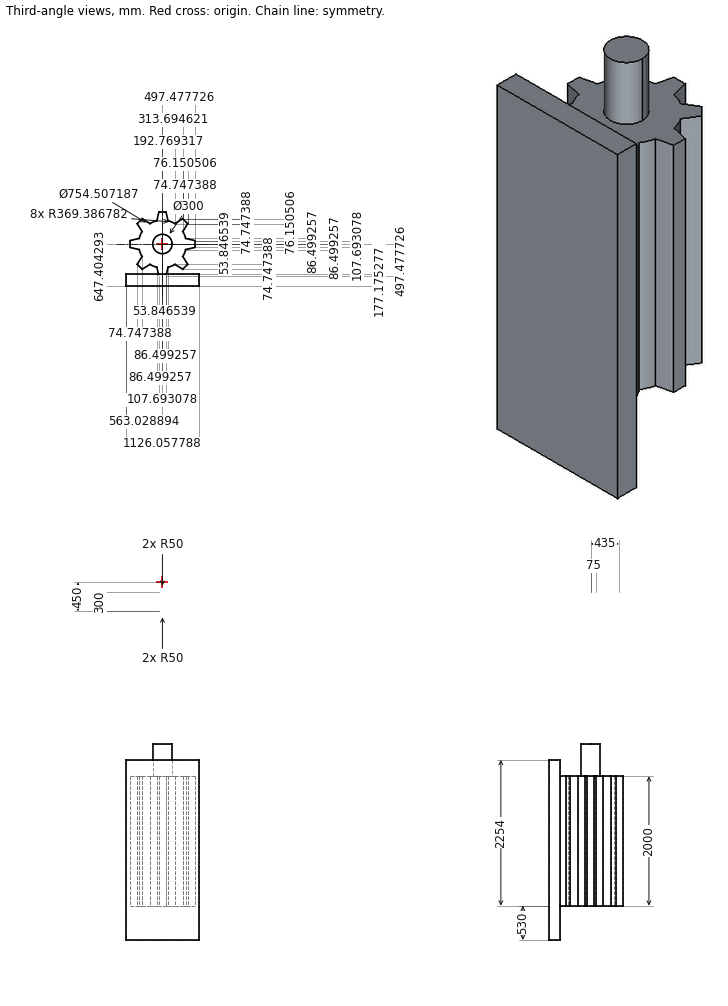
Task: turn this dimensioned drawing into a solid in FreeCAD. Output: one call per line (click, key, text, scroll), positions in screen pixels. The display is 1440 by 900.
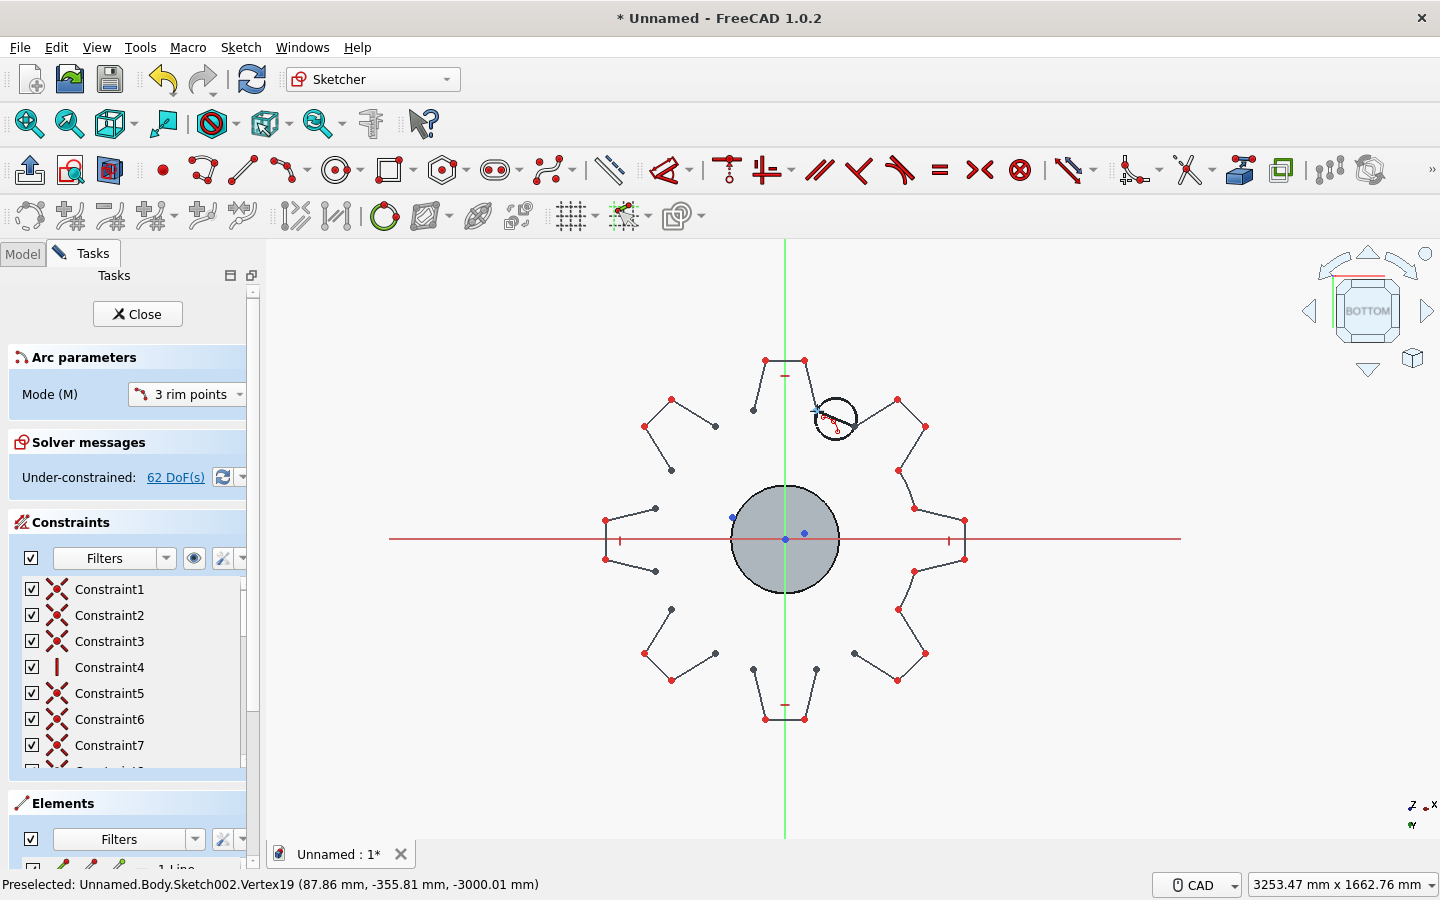
scroll(836, 416, up, 12)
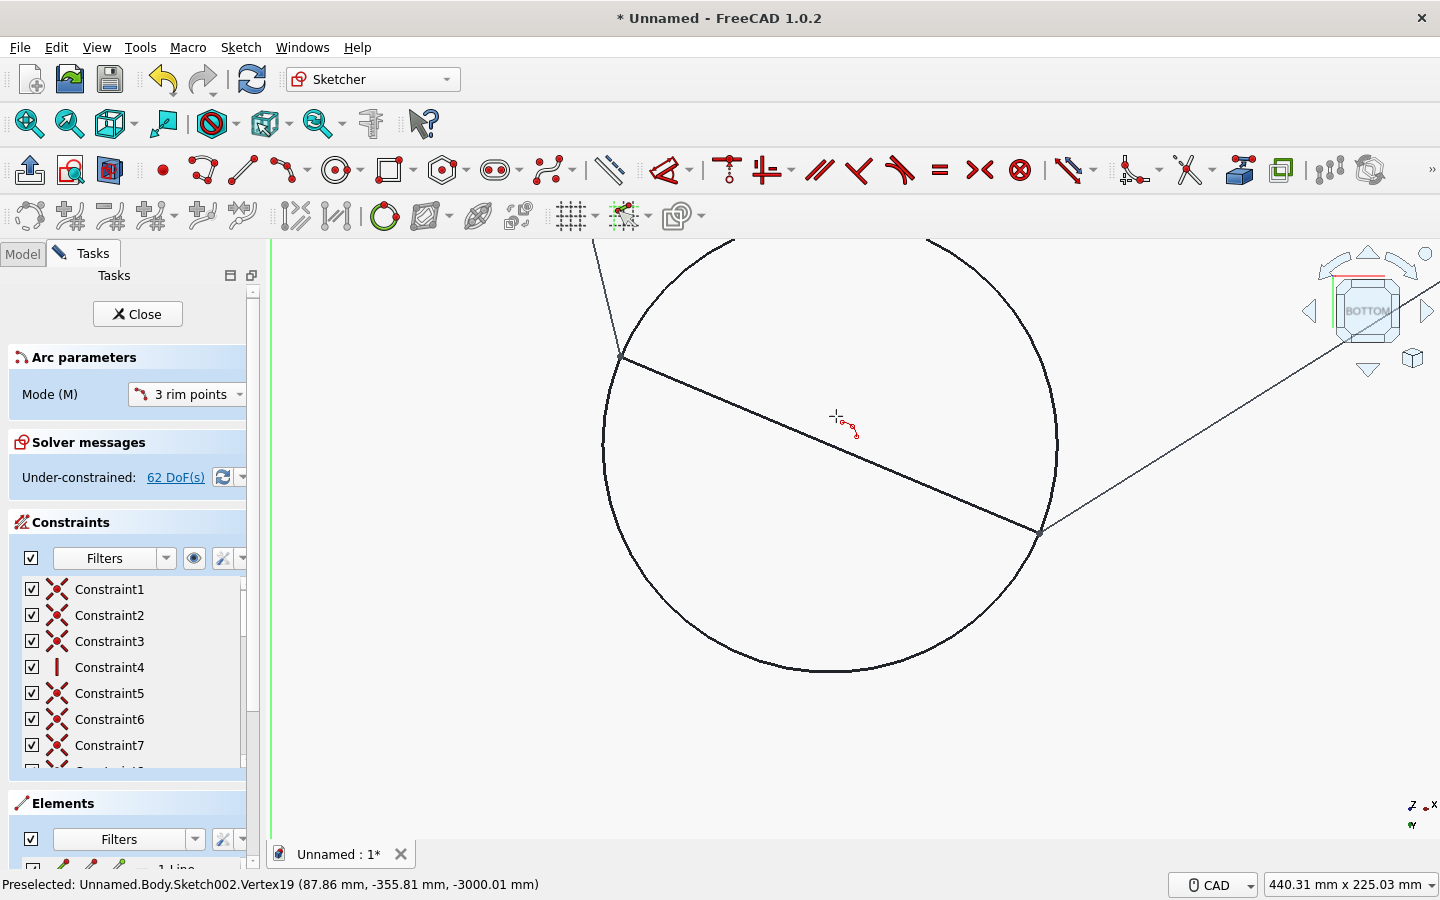
click(833, 415)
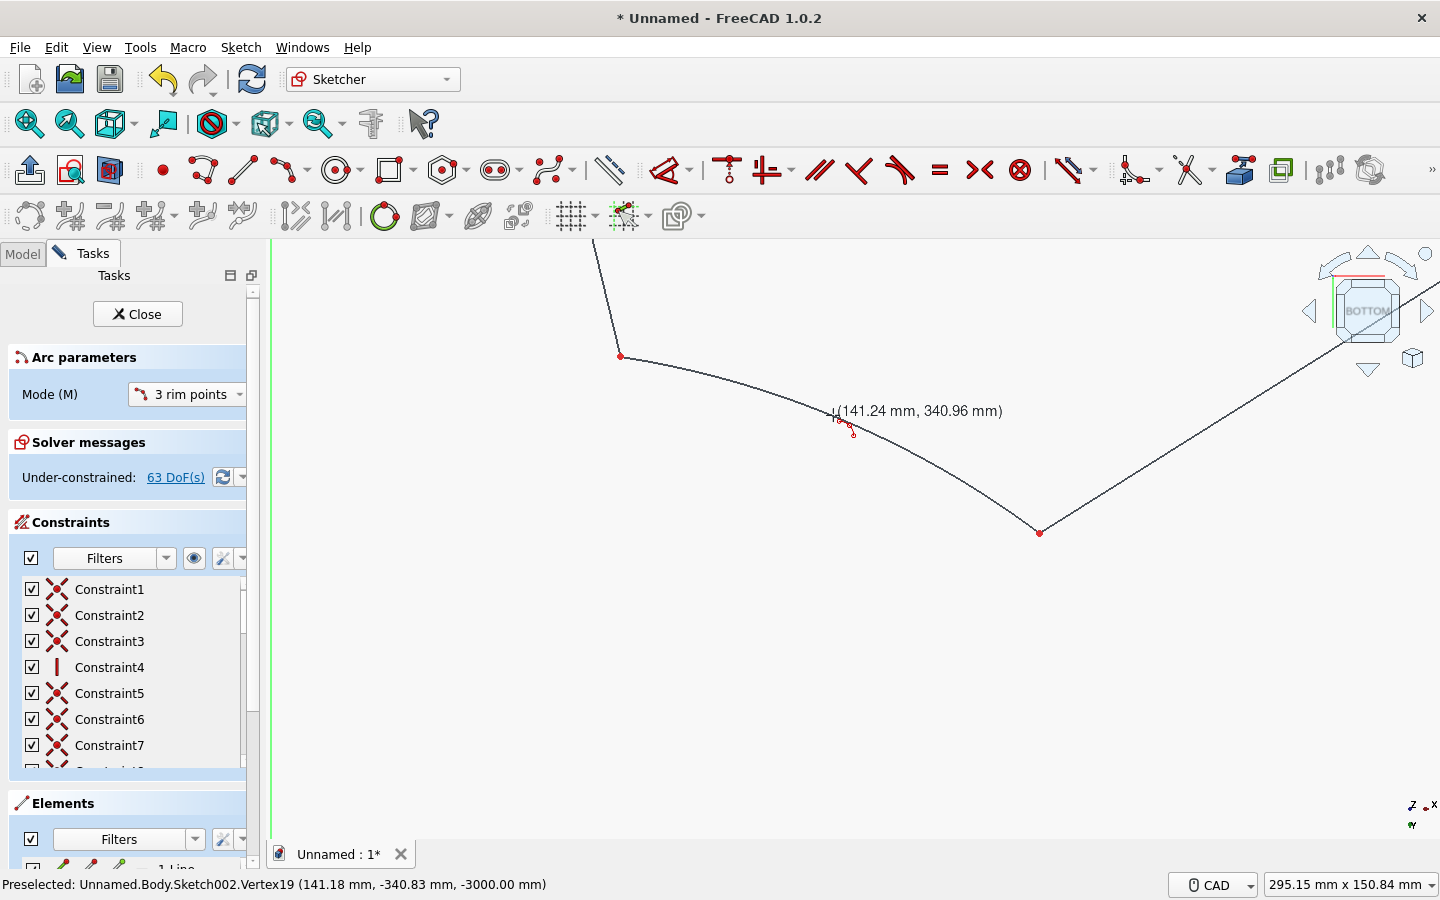
scroll(836, 416, down, 12)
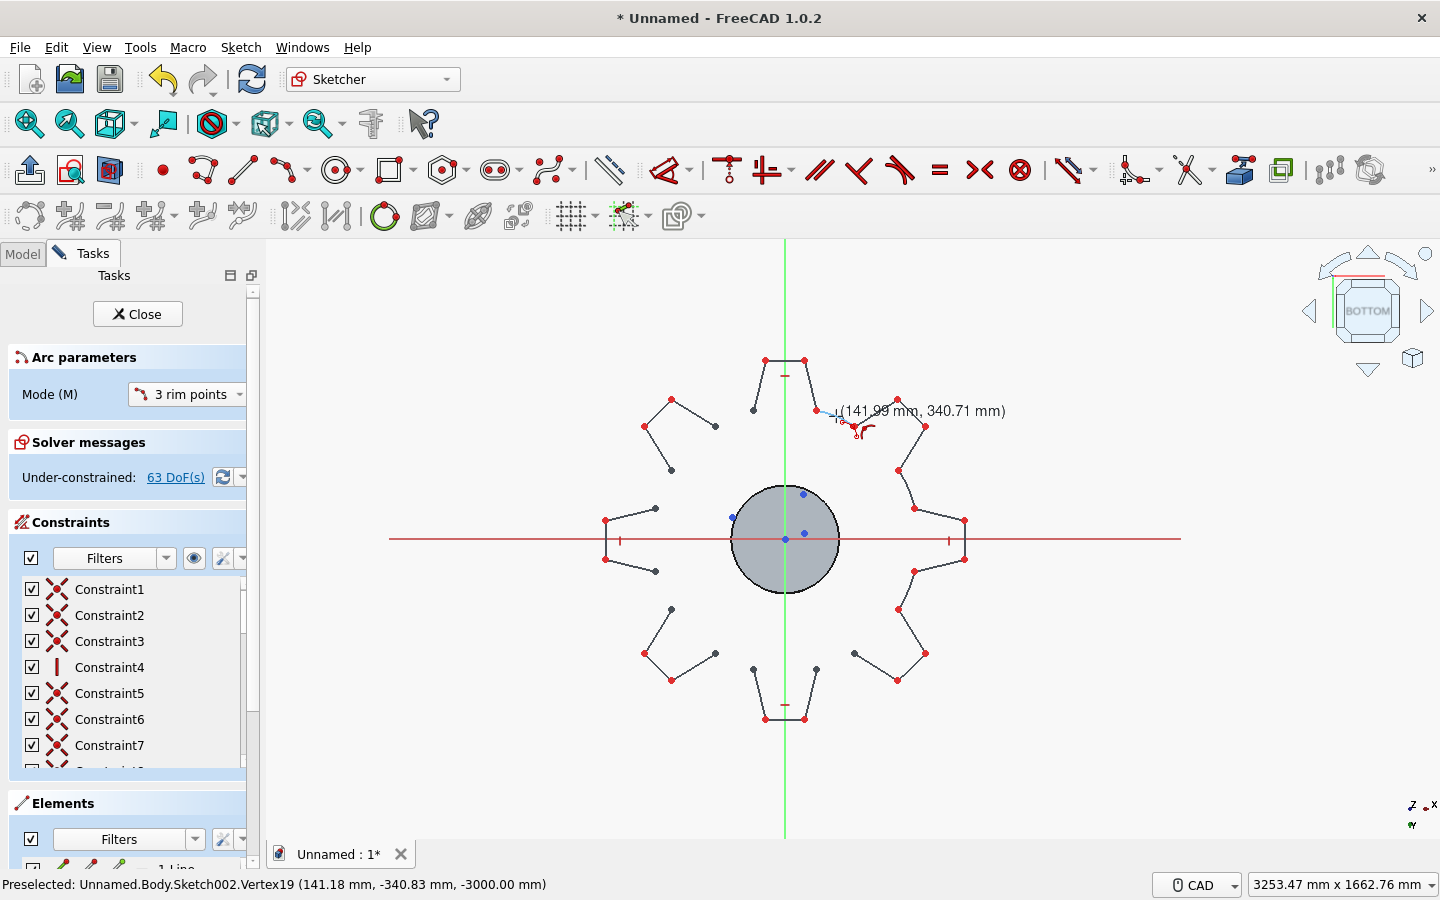
click(754, 411)
click(716, 427)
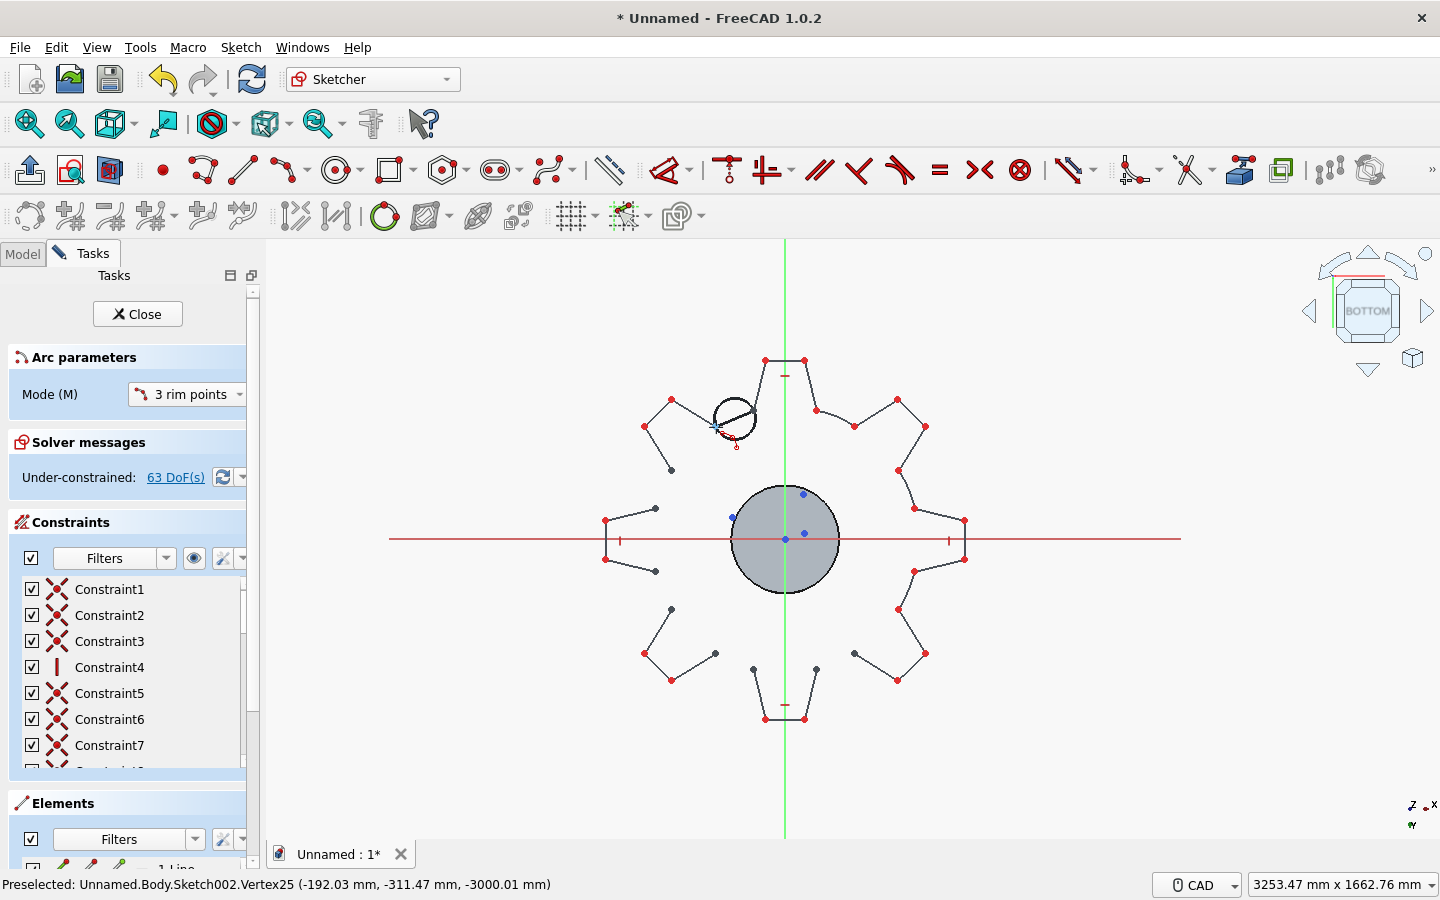
scroll(734, 416, up, 12)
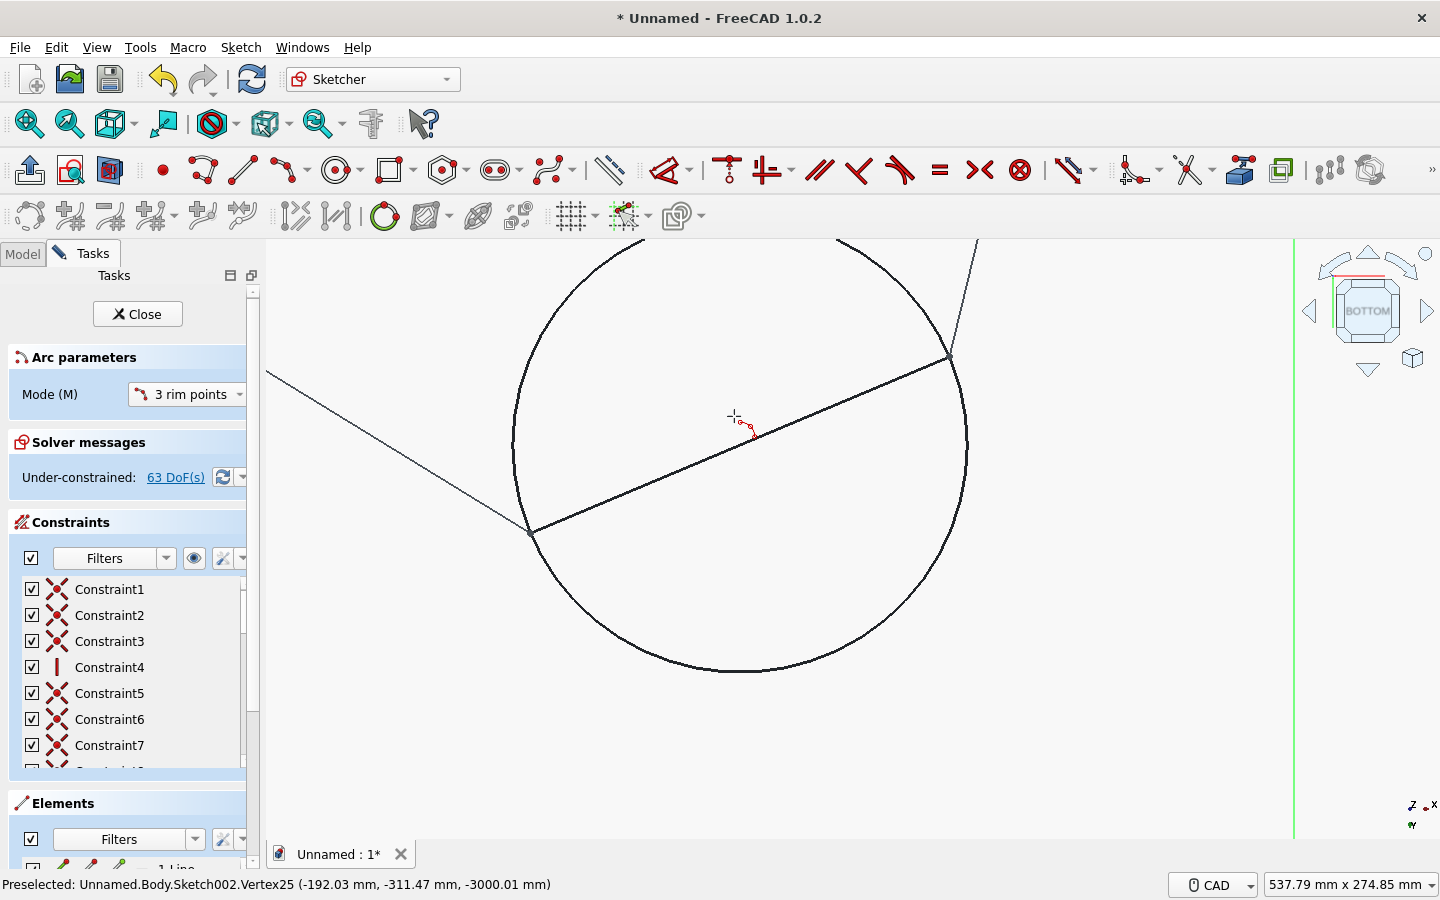
click(732, 415)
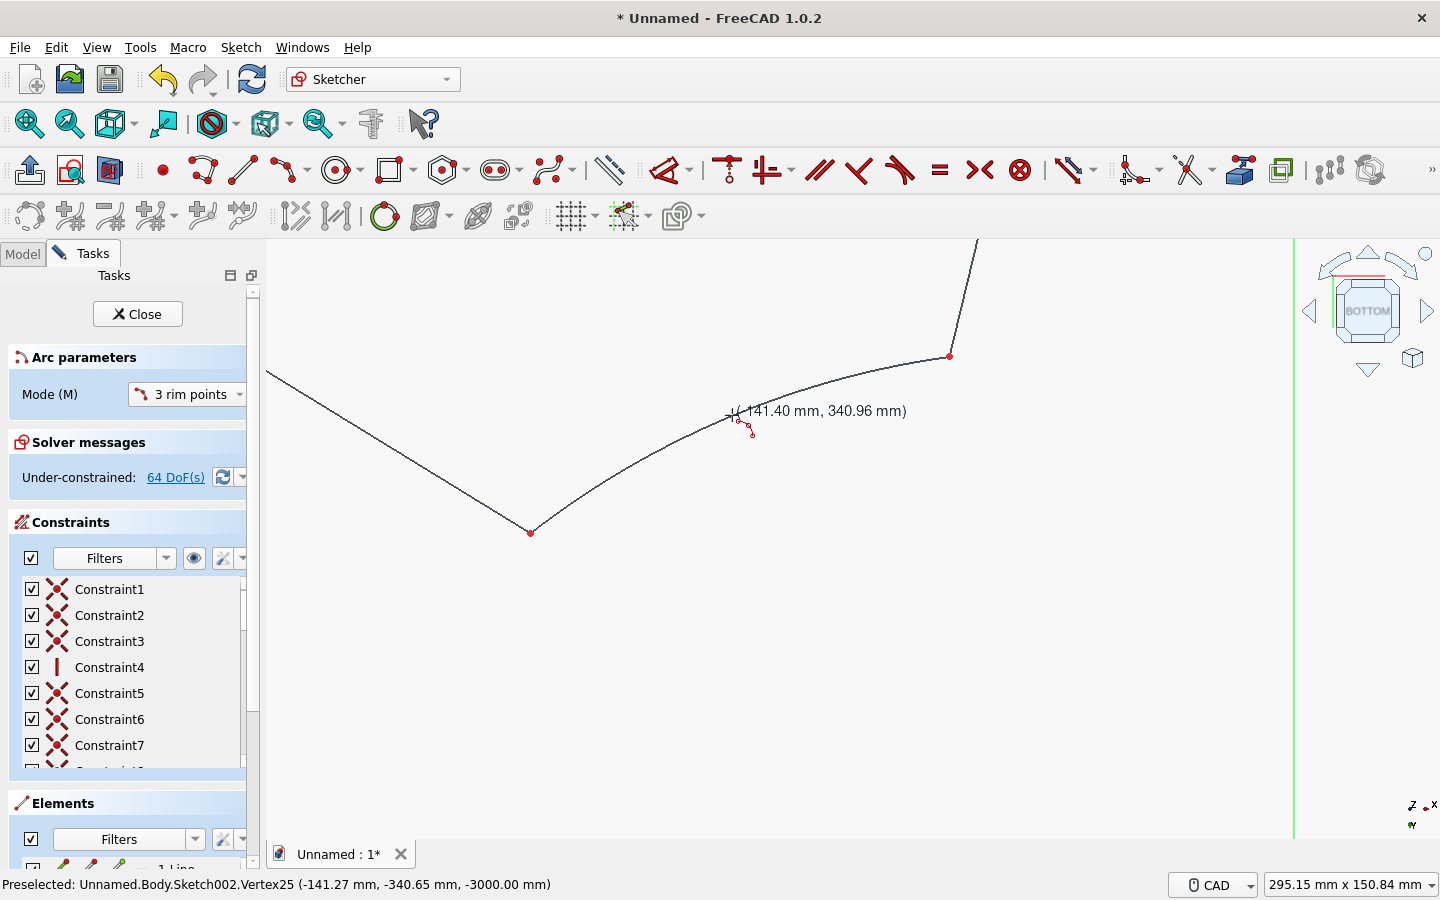
scroll(734, 416, down, 12)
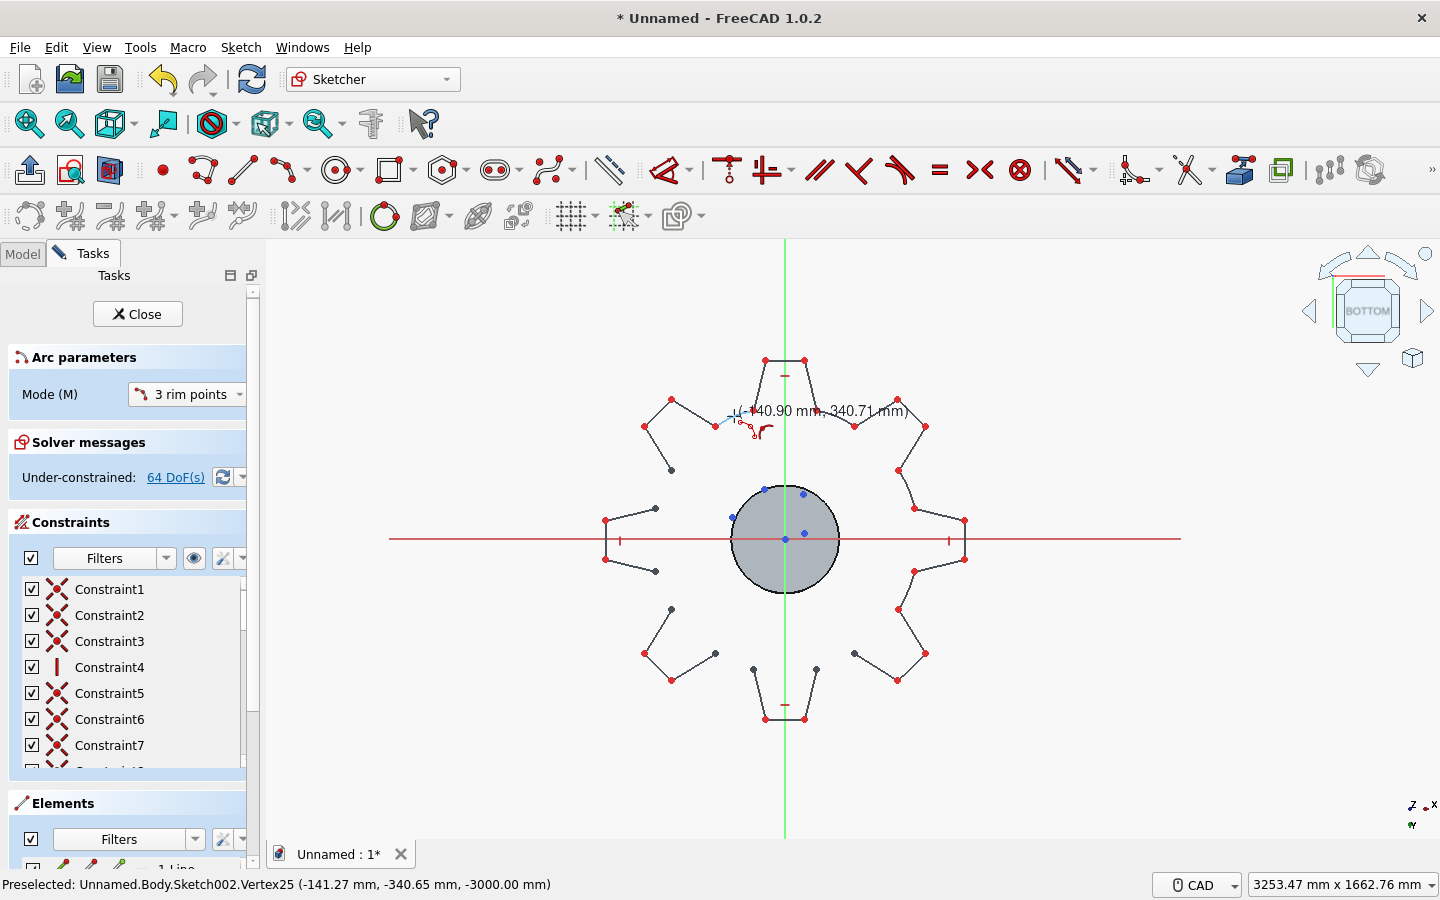
click(672, 471)
click(656, 509)